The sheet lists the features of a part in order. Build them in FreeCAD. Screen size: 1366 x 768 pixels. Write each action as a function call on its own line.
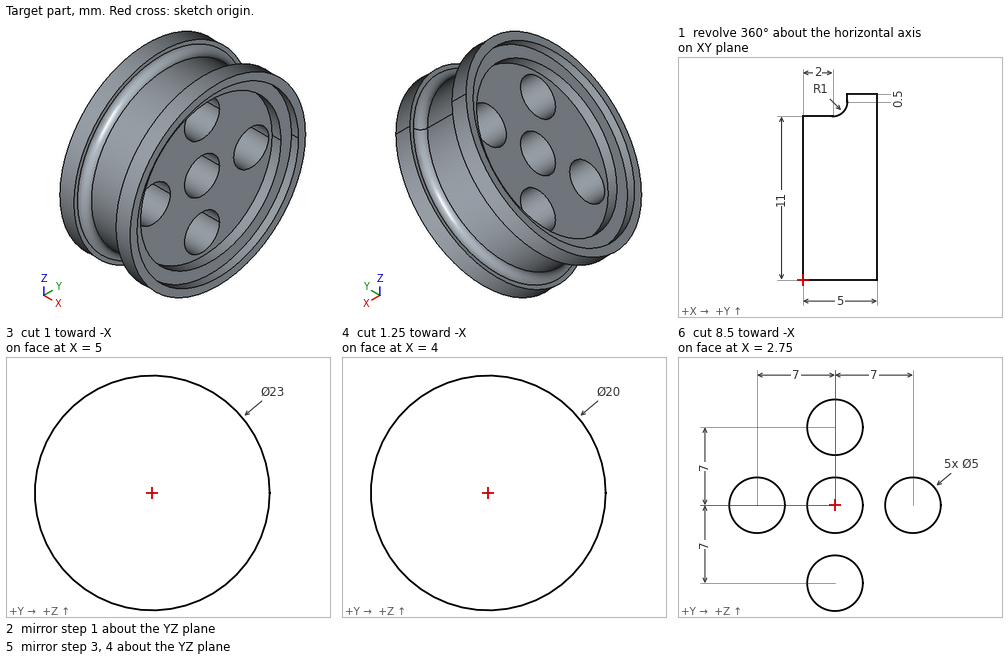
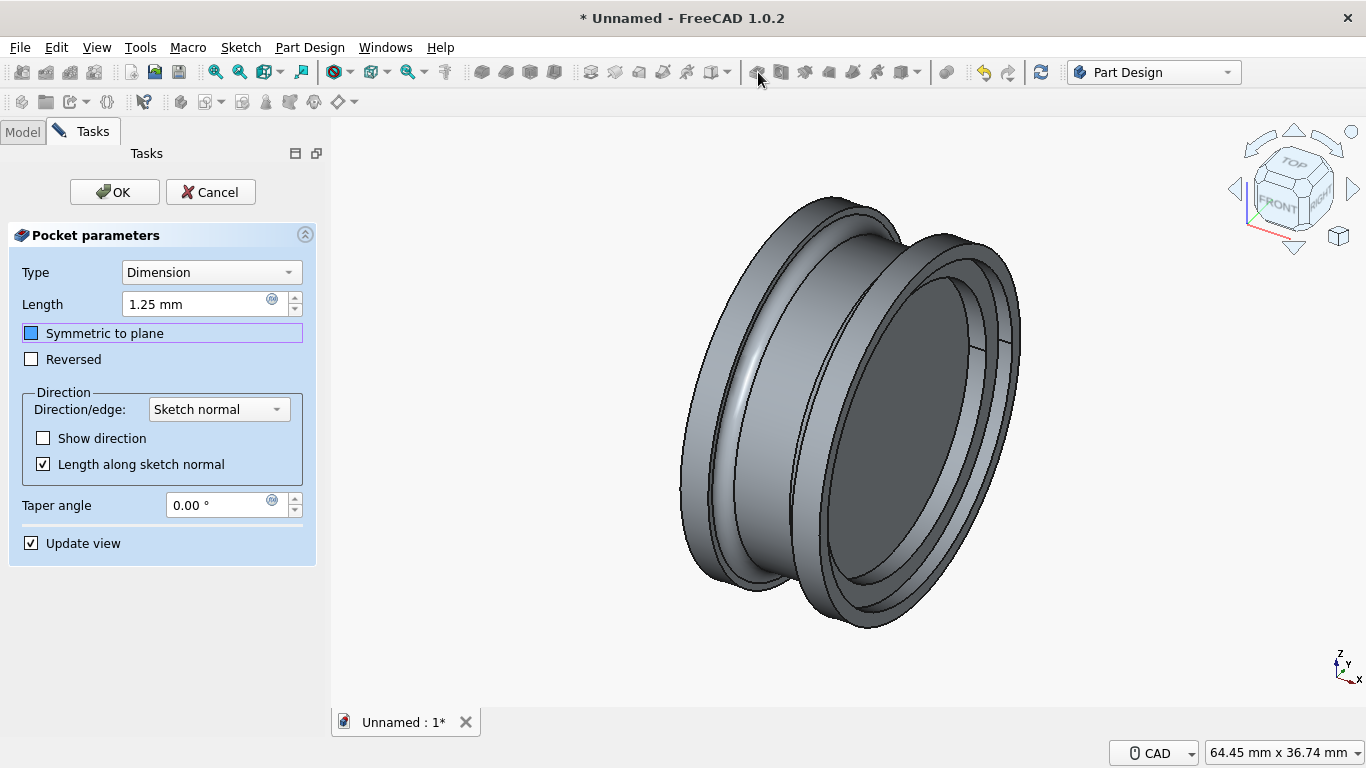
click(115, 192)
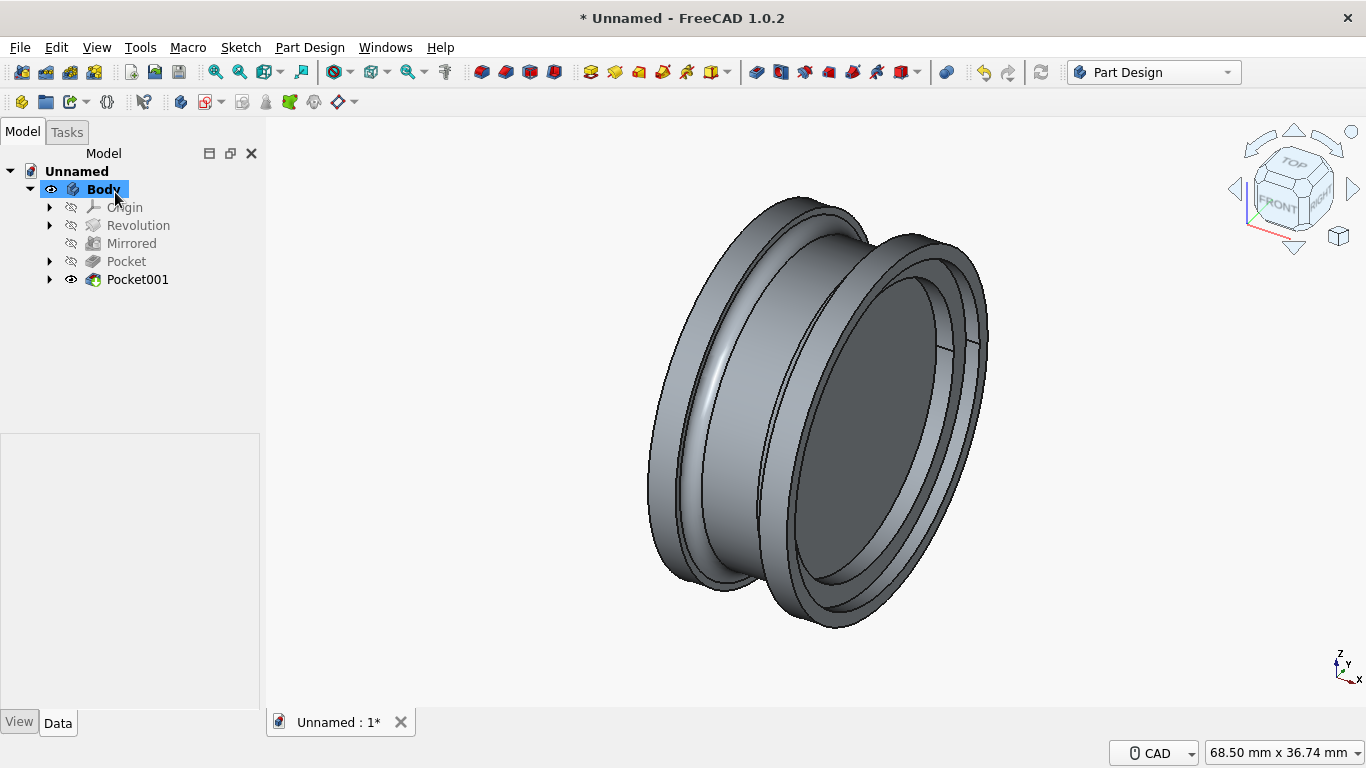
click(116, 261)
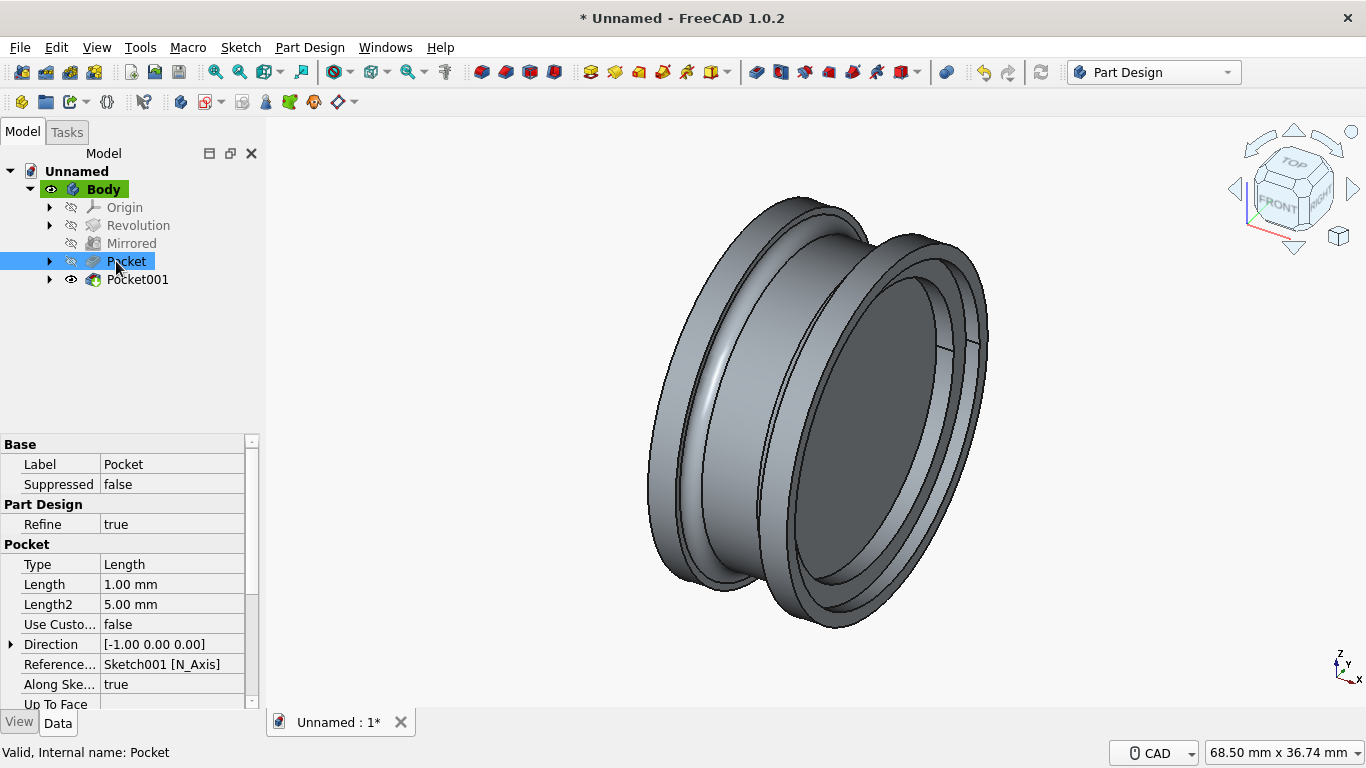
click(116, 279, ctrl)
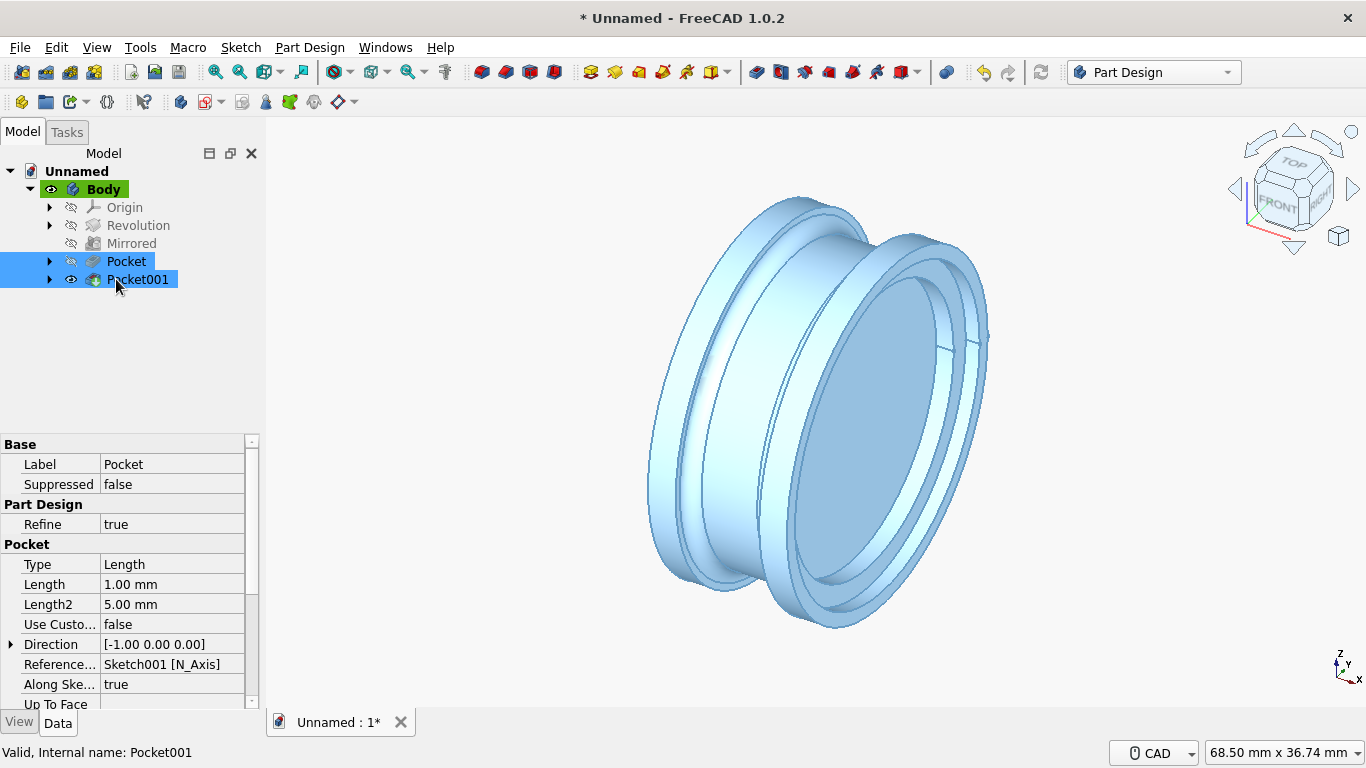
click(22, 72)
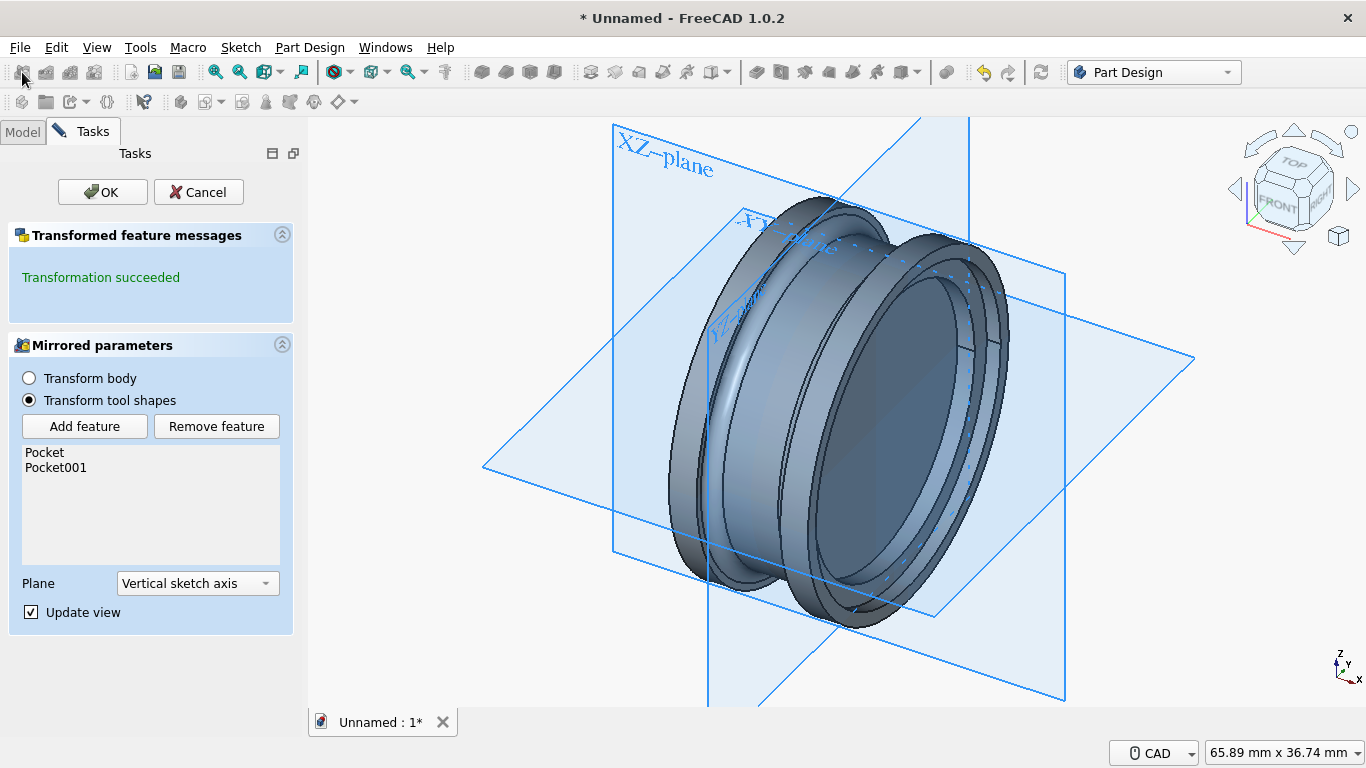
click(198, 584)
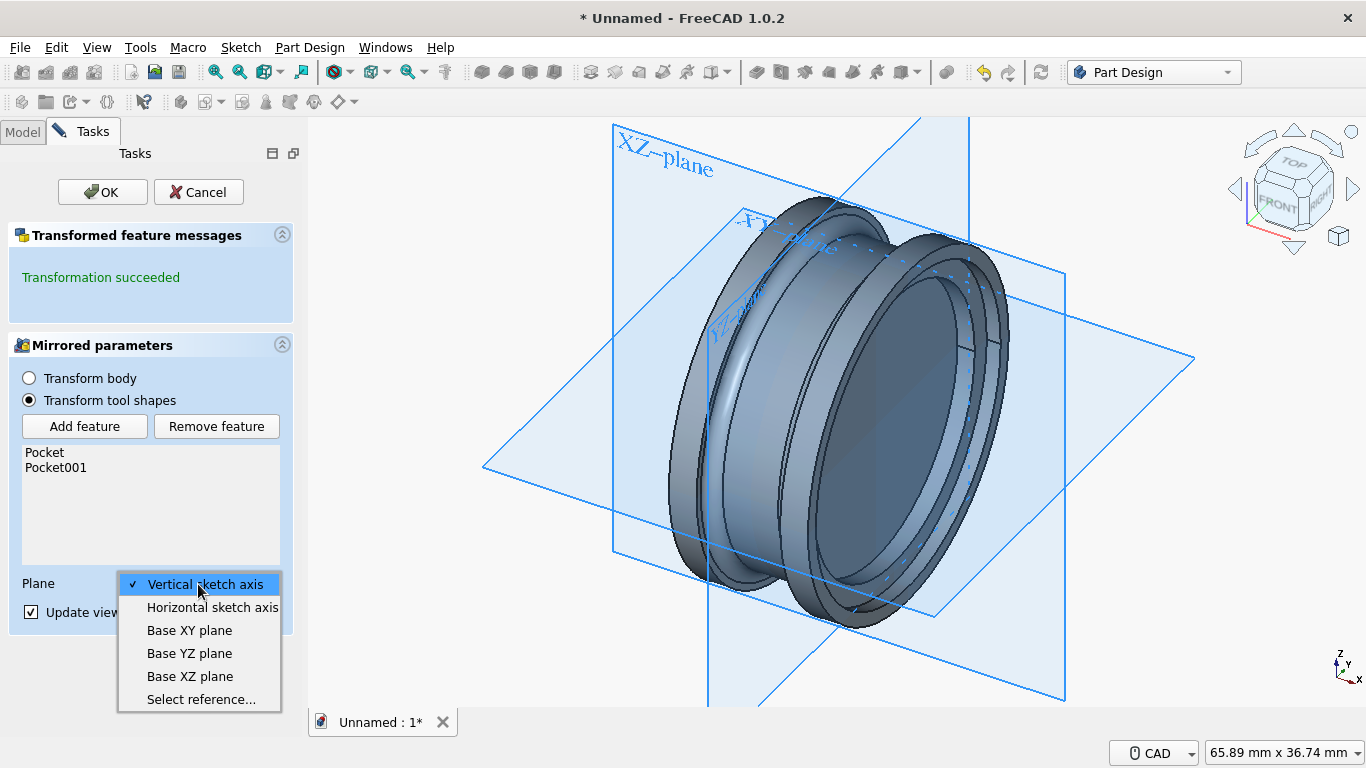
click(198, 654)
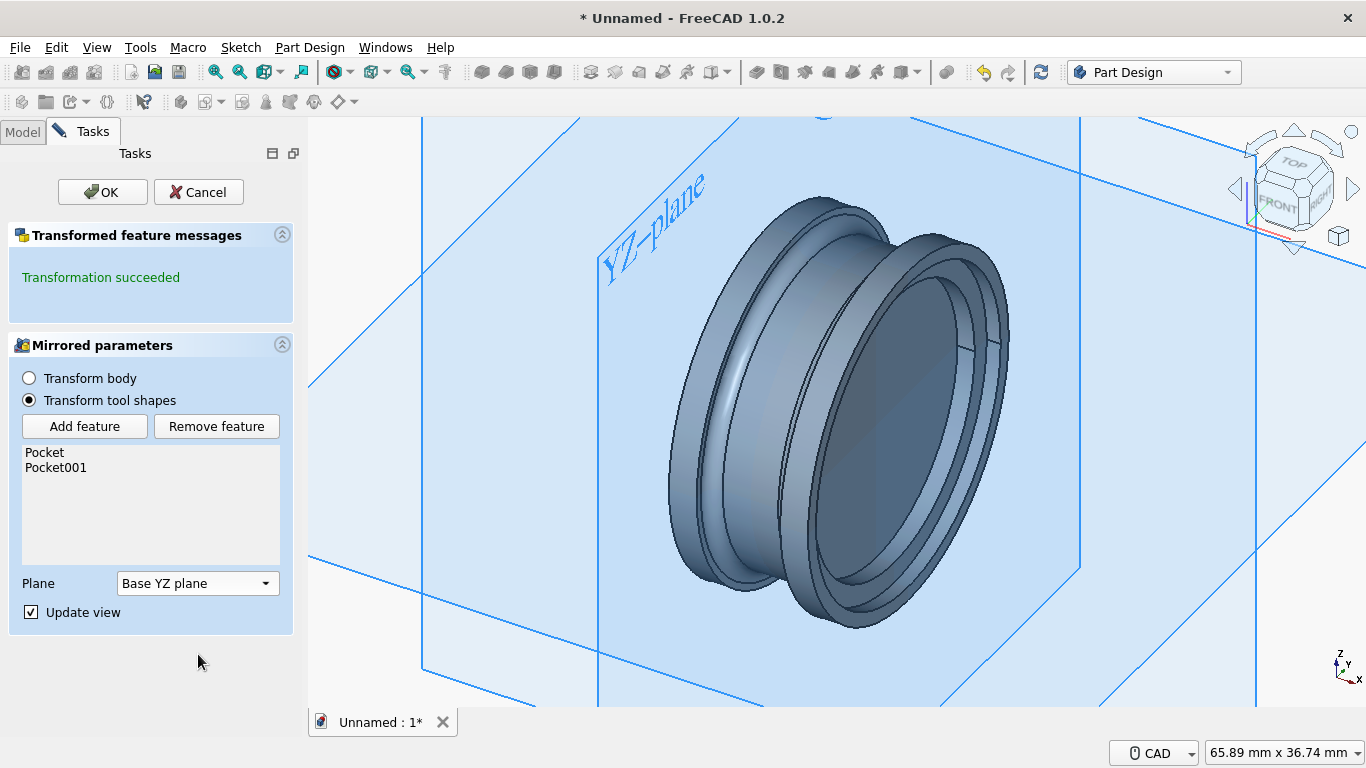
click(103, 192)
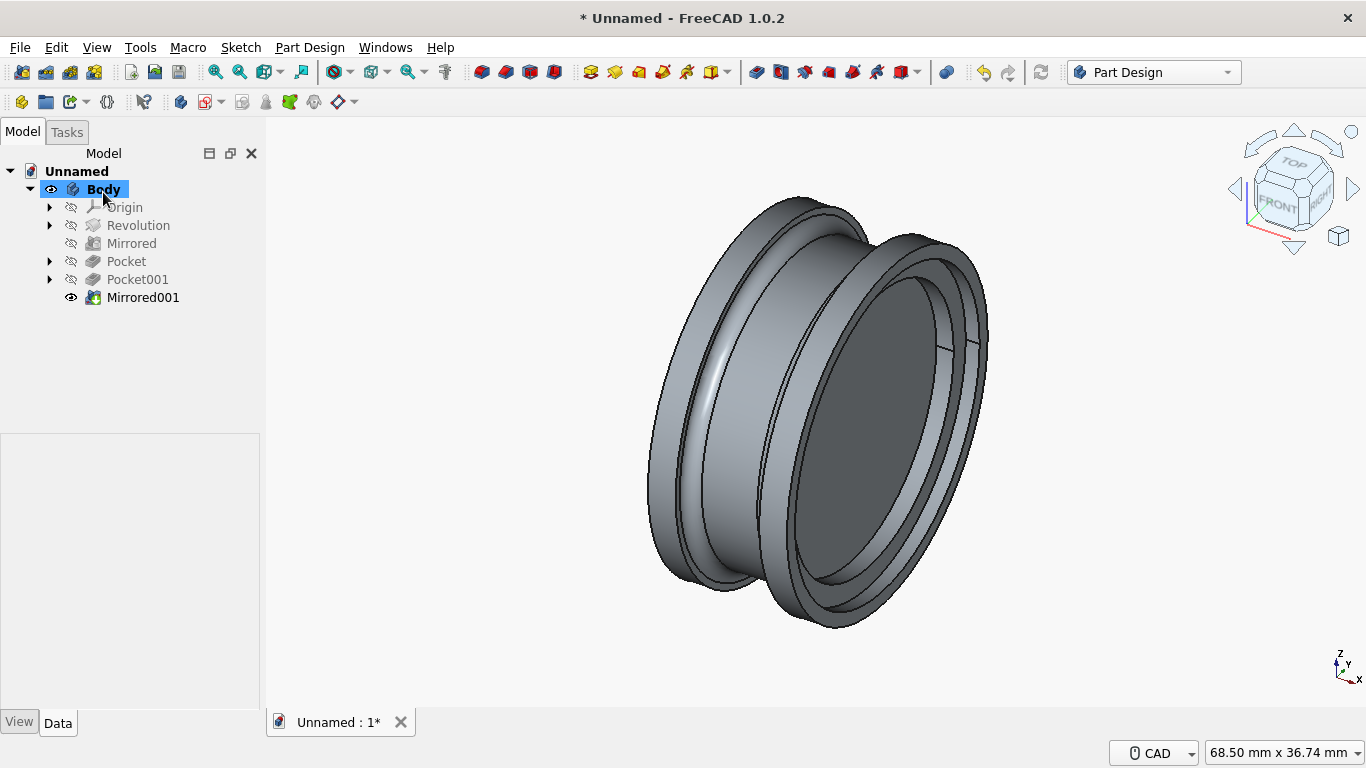
click(856, 424)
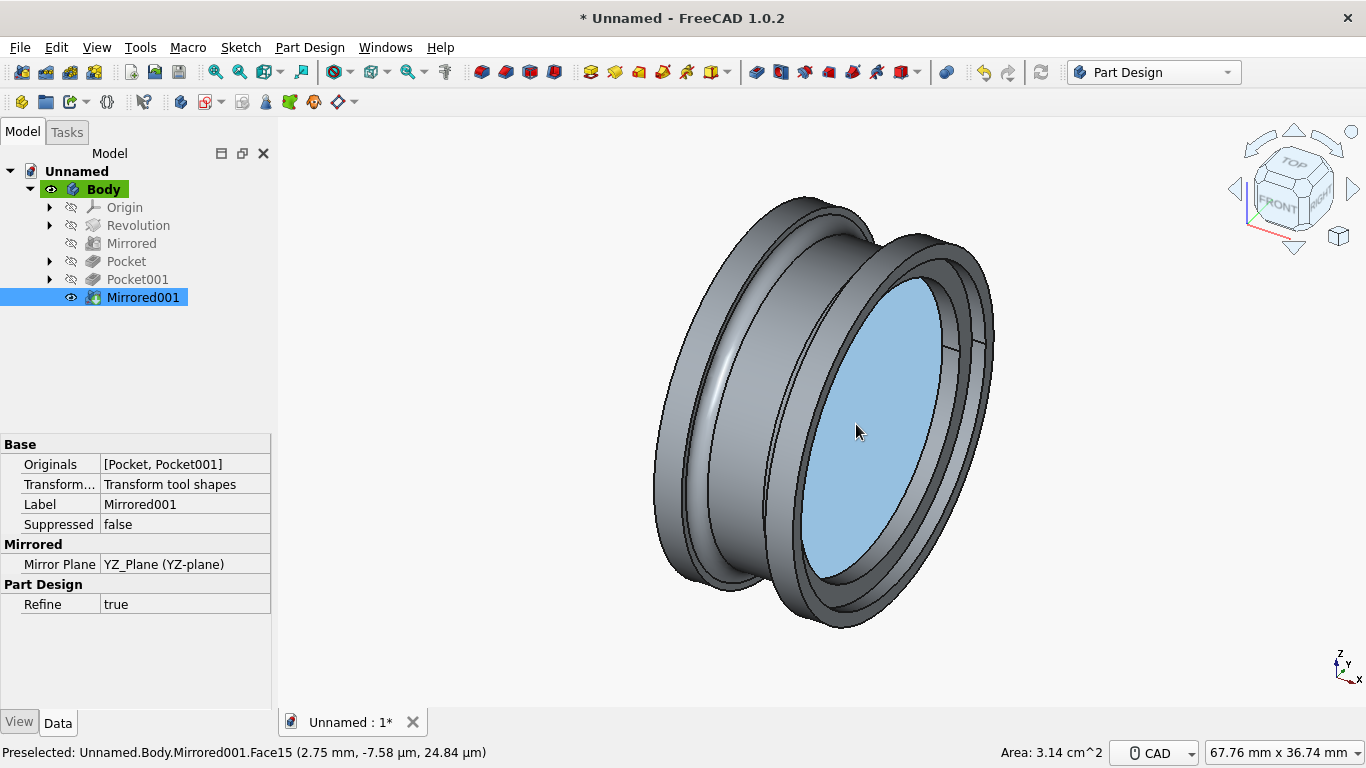
click(206, 102)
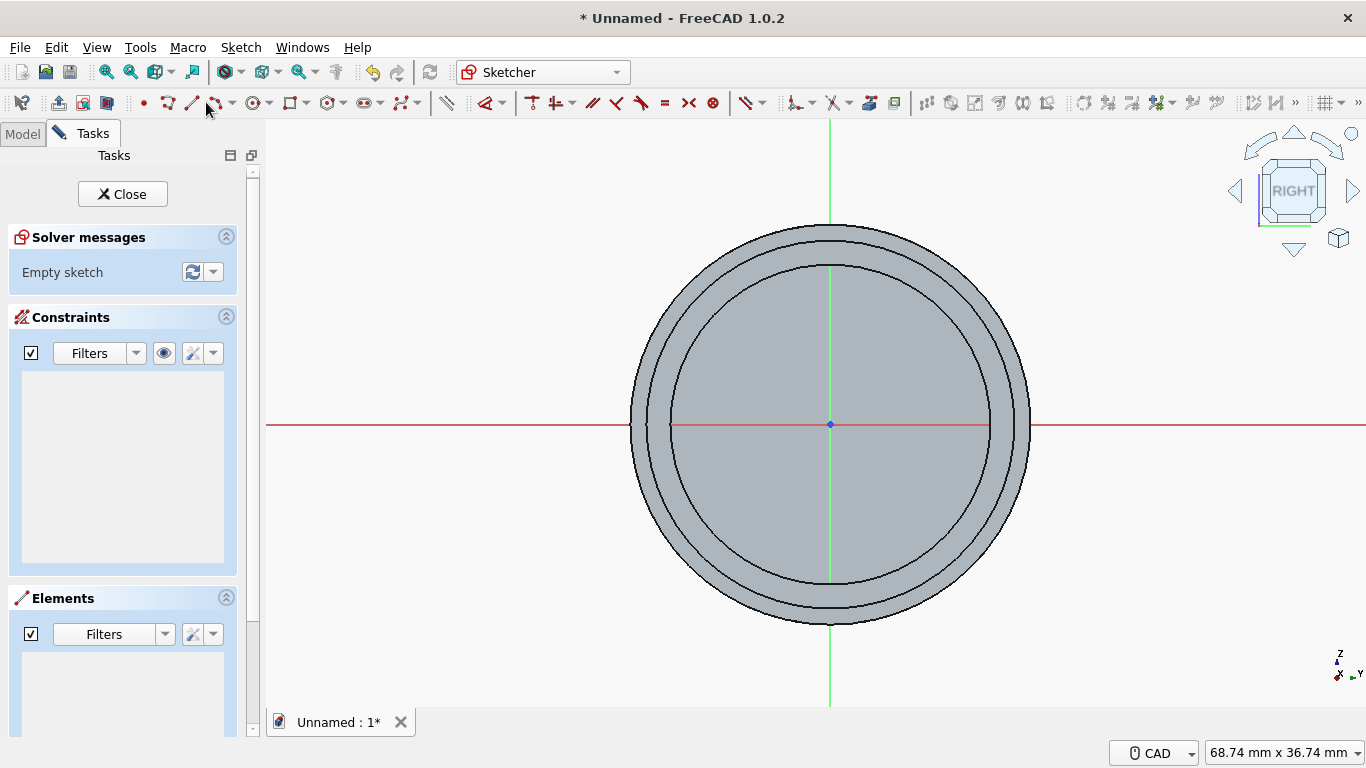
click(108, 104)